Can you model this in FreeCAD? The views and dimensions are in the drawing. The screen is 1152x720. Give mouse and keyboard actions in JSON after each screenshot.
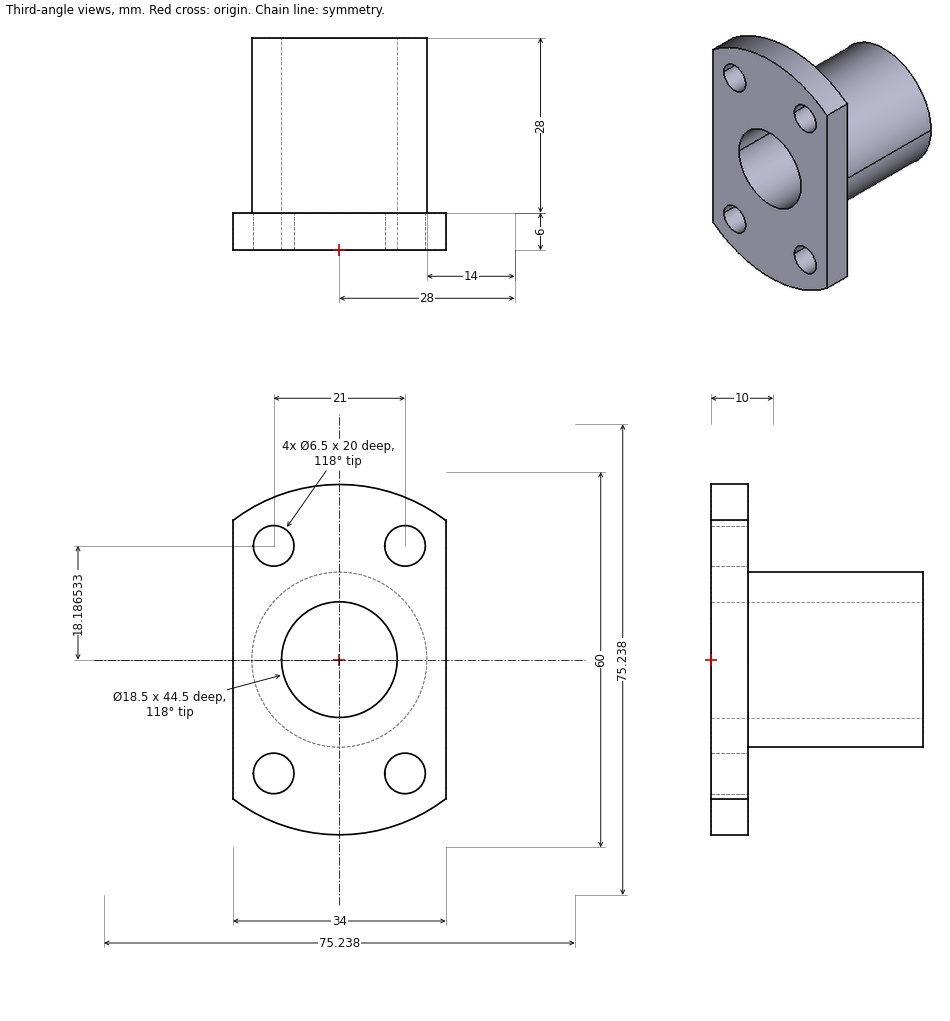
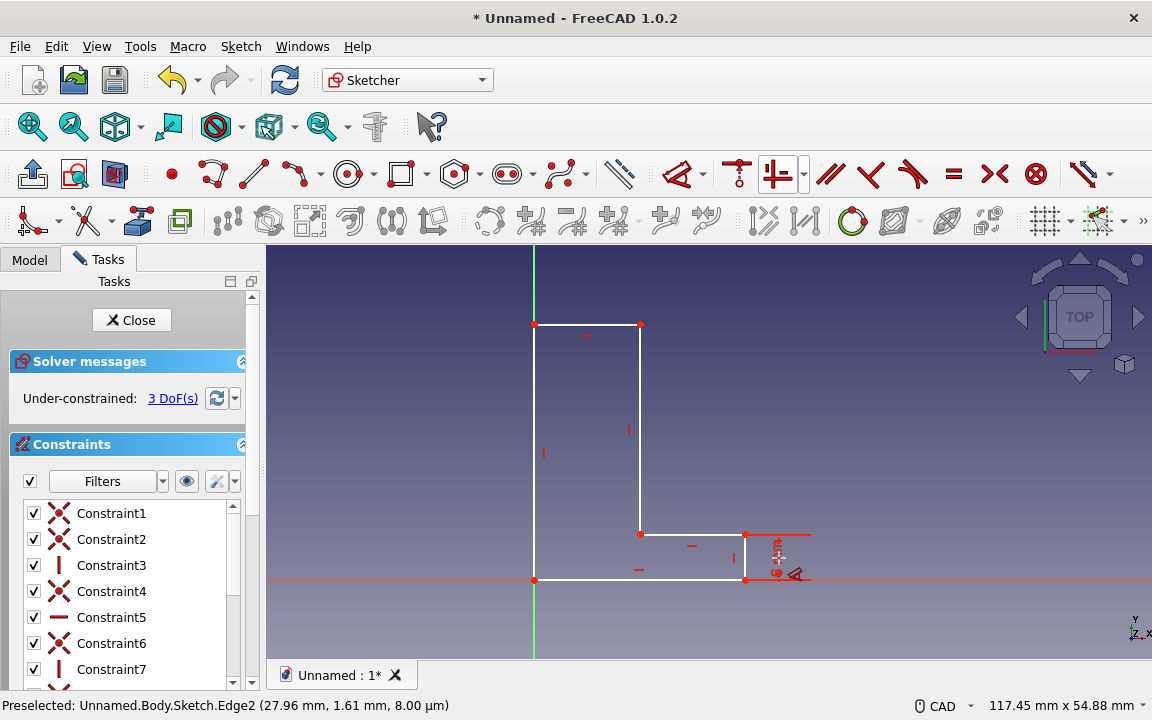
{"action": "left_click", "coordinate": [597, 580]}
{"action": "left_click", "coordinate": [640, 614]}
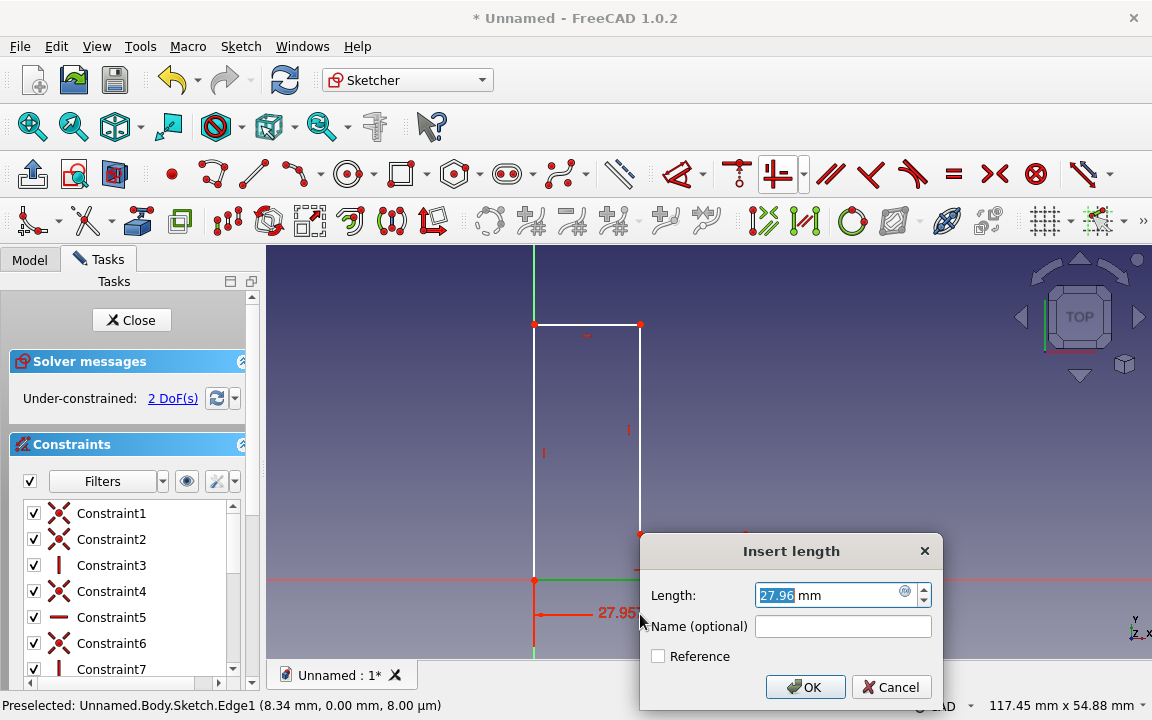
{"action": "type", "text": "28"}
{"action": "key", "text": "Return"}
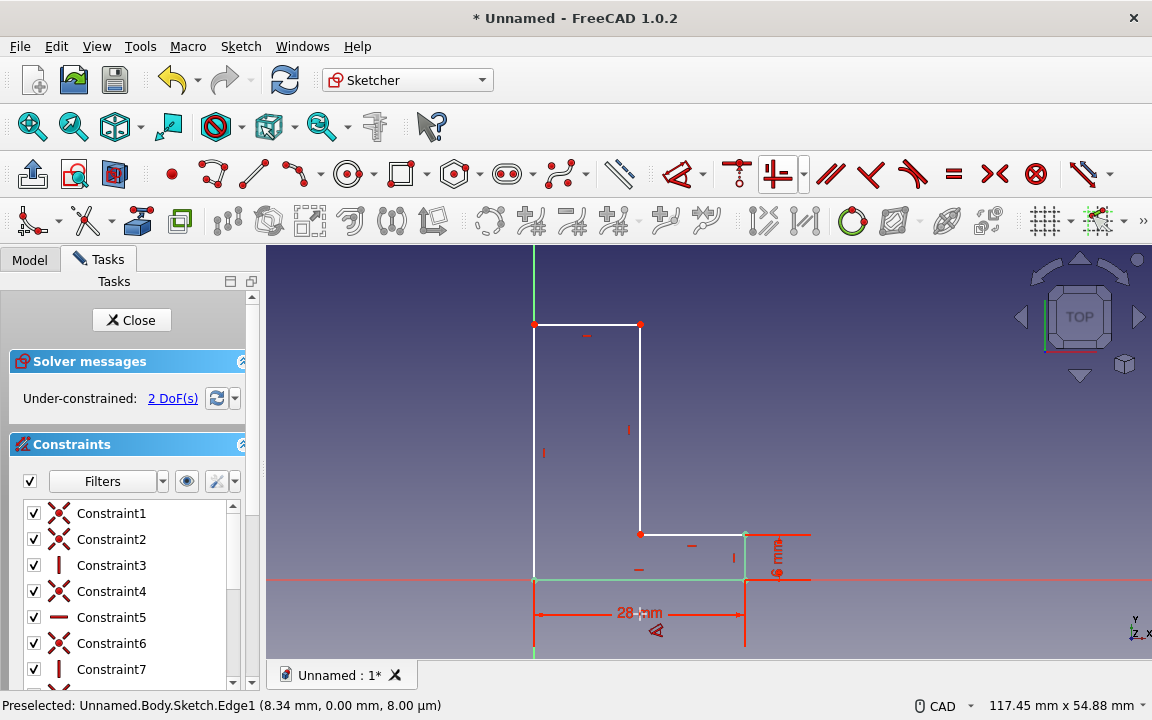
{"action": "left_click", "coordinate": [714, 535]}
{"action": "left_click", "coordinate": [693, 501]}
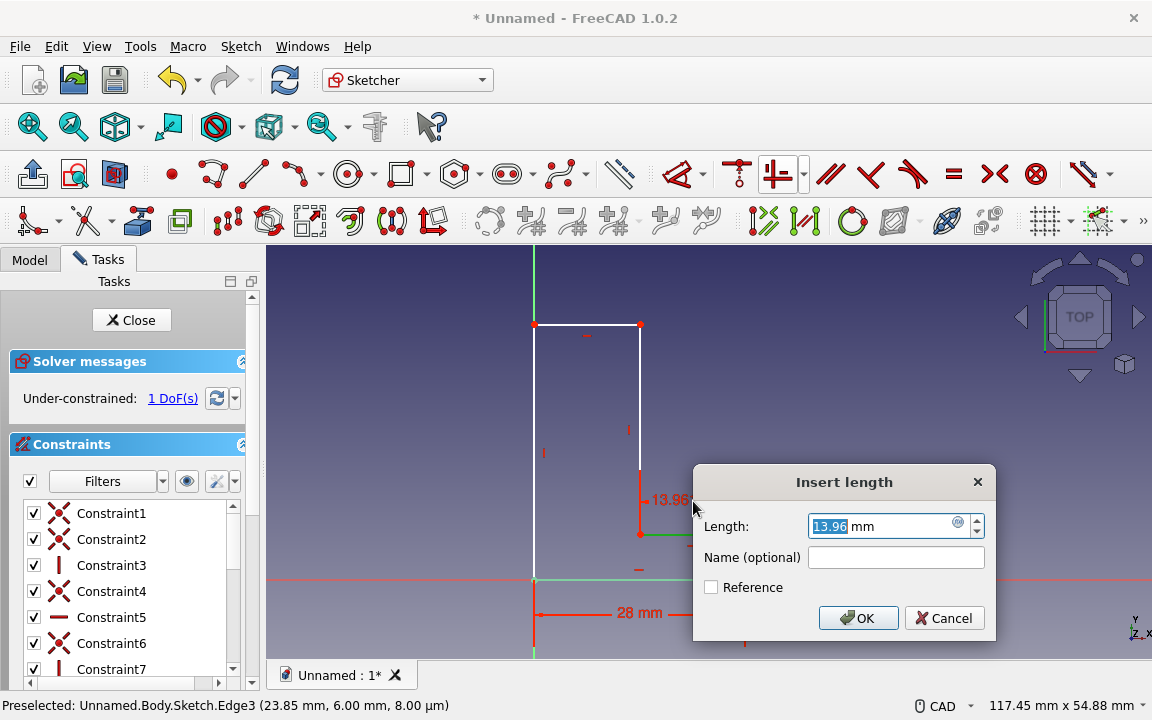
{"action": "type", "text": "14"}
{"action": "key", "text": "Return"}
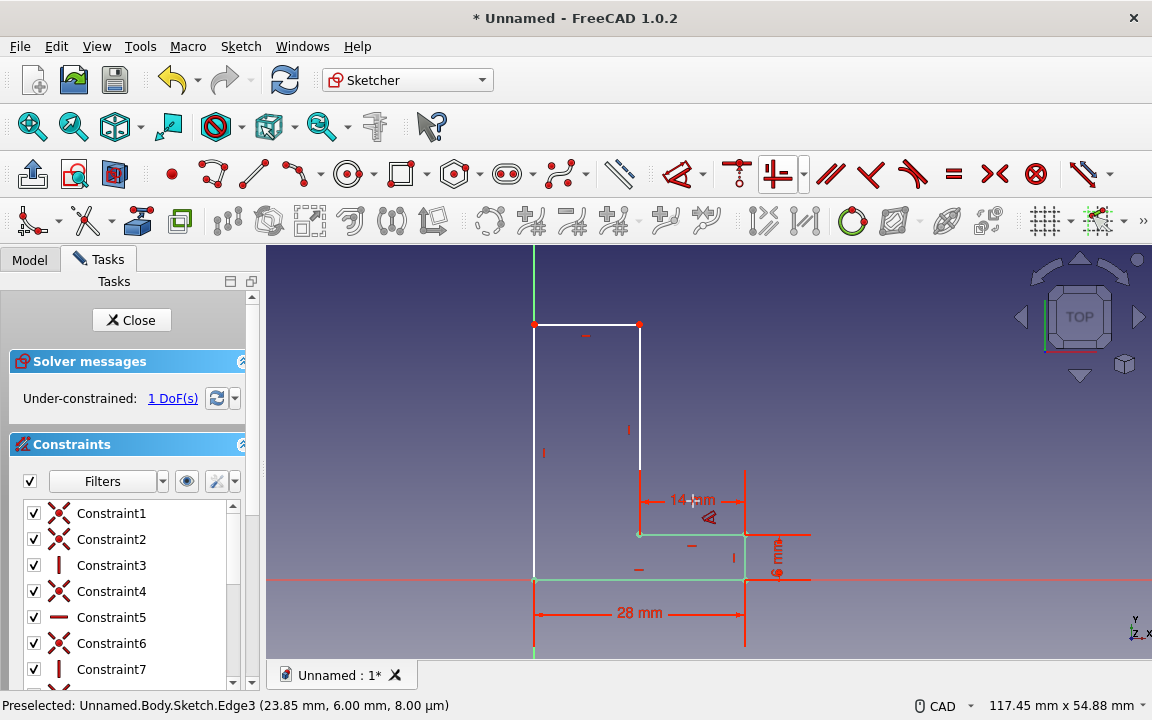
{"action": "left_click", "coordinate": [640, 472]}
{"action": "left_click", "coordinate": [674, 430]}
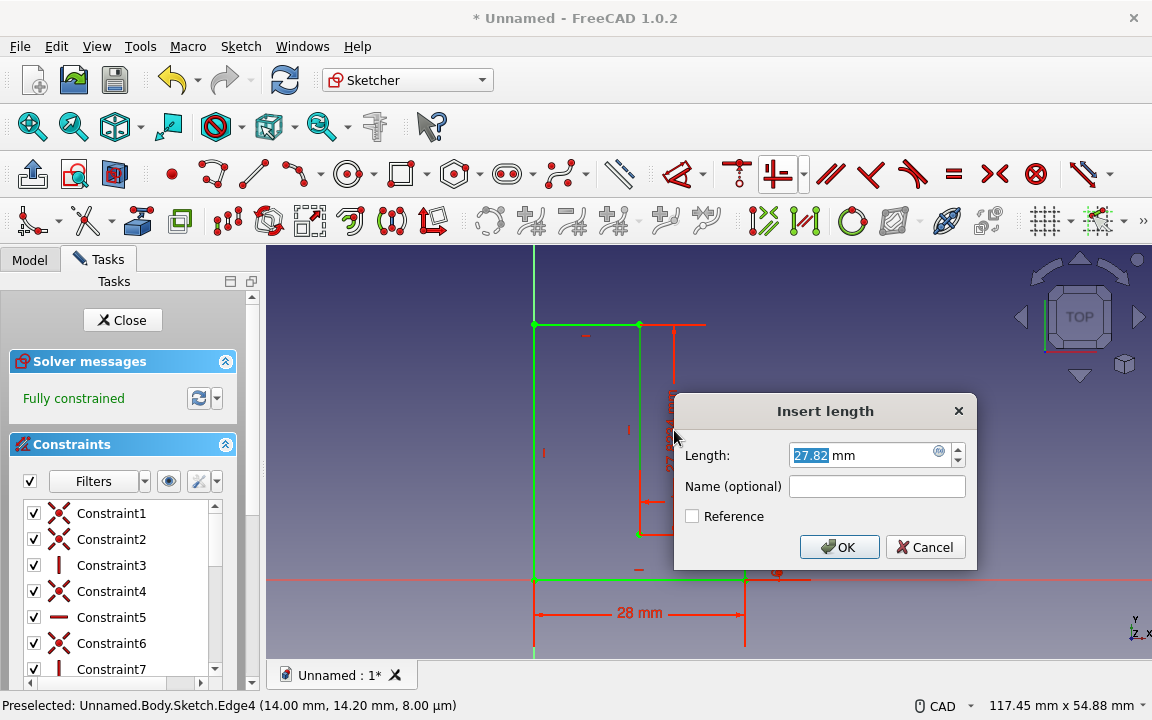
{"action": "type", "text": "28"}
{"action": "key", "text": "Return"}
{"action": "key", "text": "Escape"}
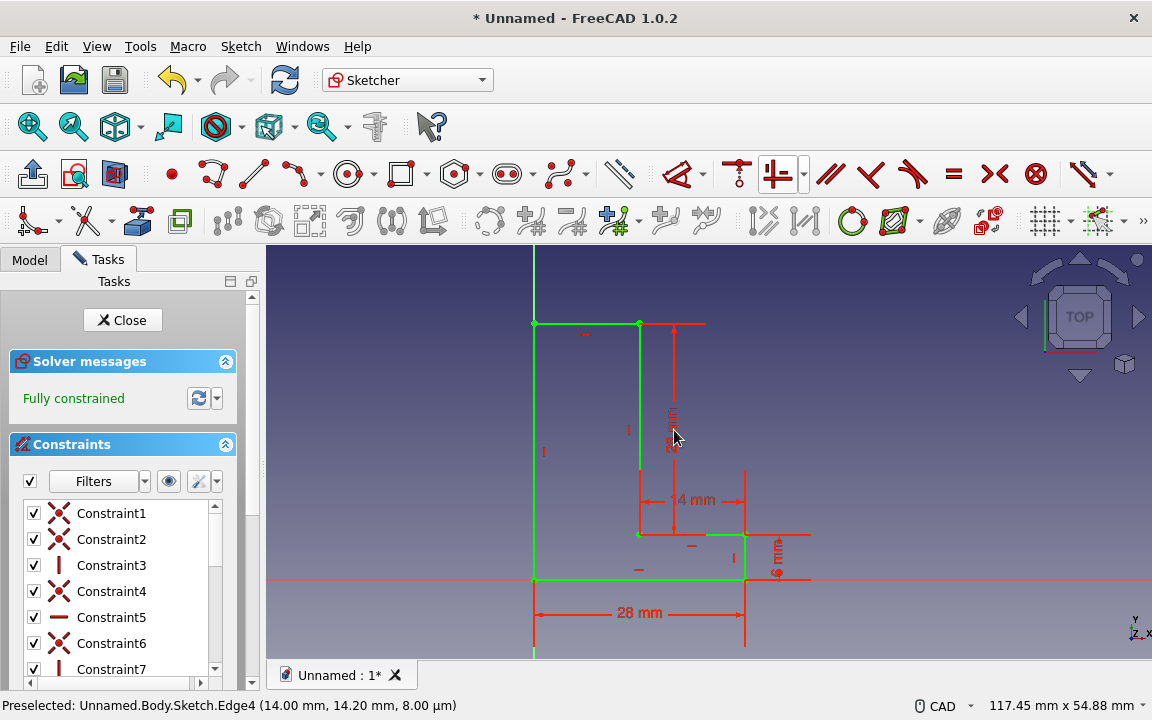
{"action": "left_click", "coordinate": [123, 320]}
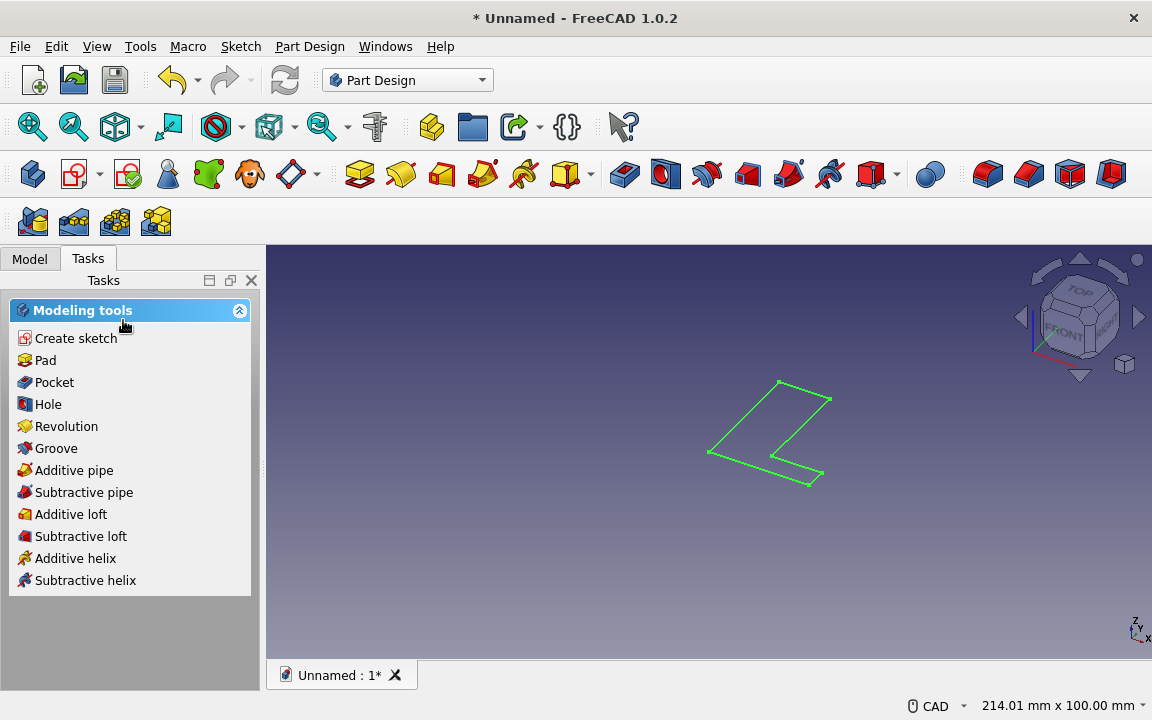
{"action": "left_click", "coordinate": [401, 174]}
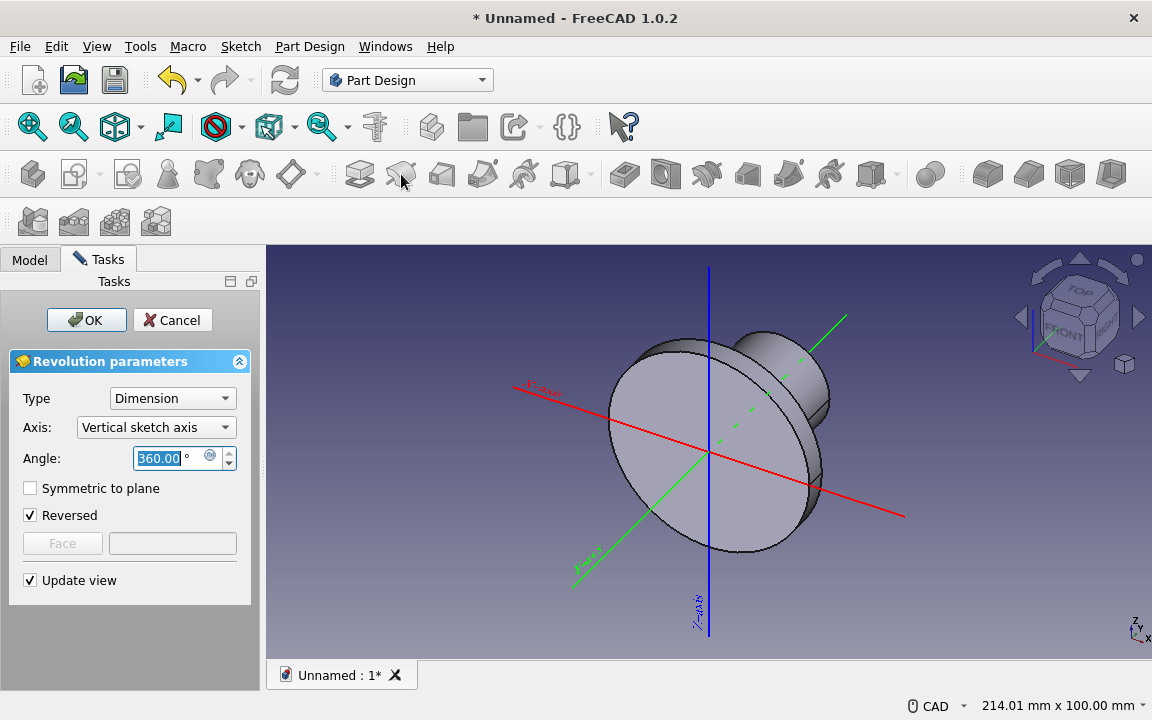
{"action": "left_click", "coordinate": [87, 320]}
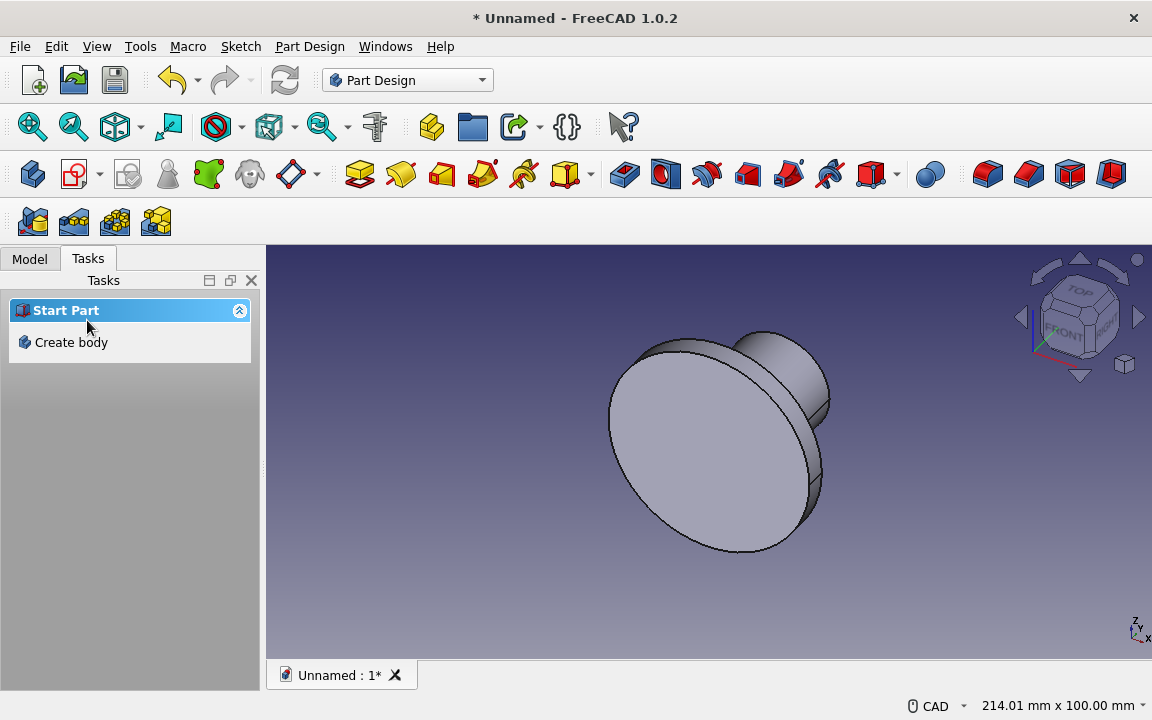
{"action": "left_click", "coordinate": [74, 174]}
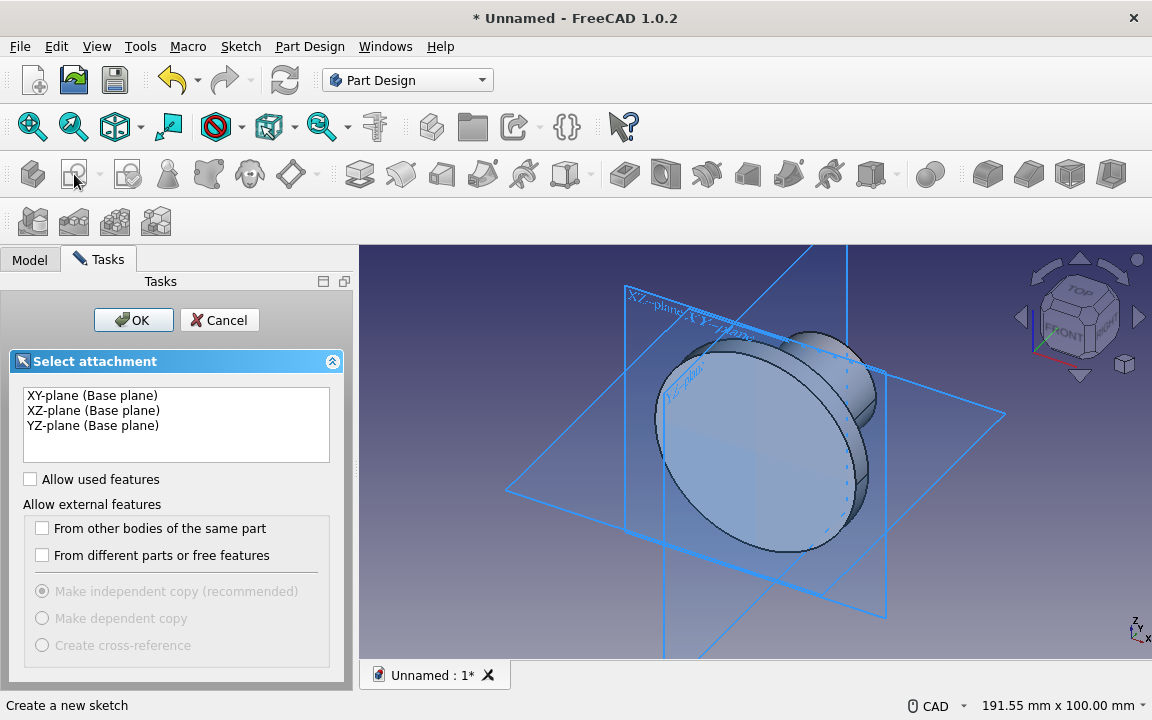
{"action": "left_click", "coordinate": [84, 410]}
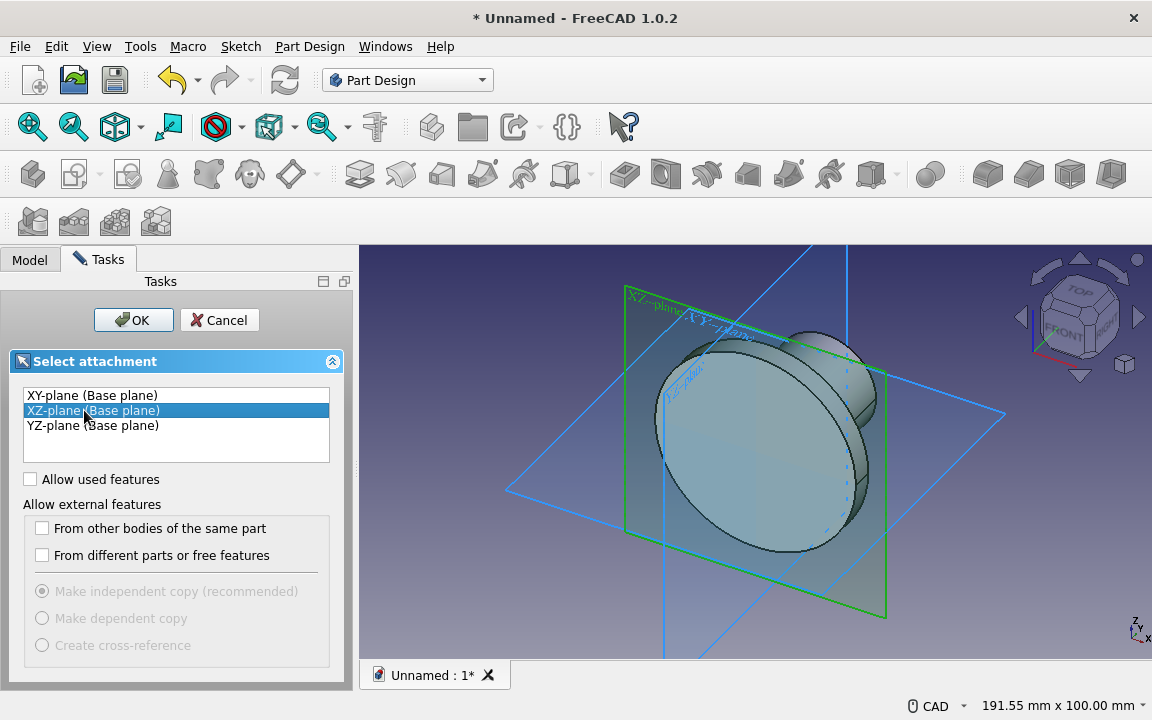
{"action": "left_click", "coordinate": [134, 320]}